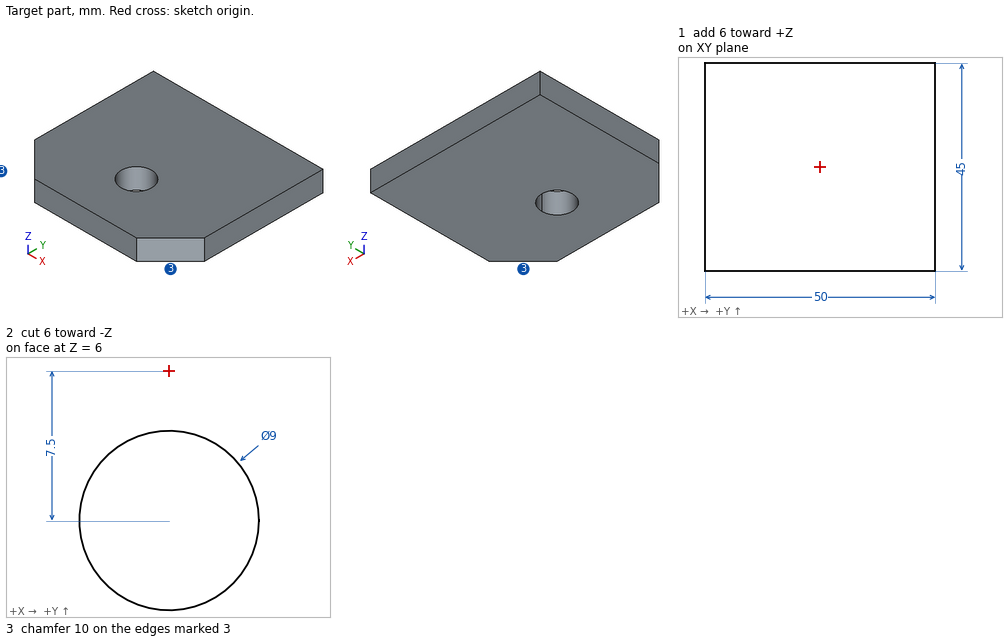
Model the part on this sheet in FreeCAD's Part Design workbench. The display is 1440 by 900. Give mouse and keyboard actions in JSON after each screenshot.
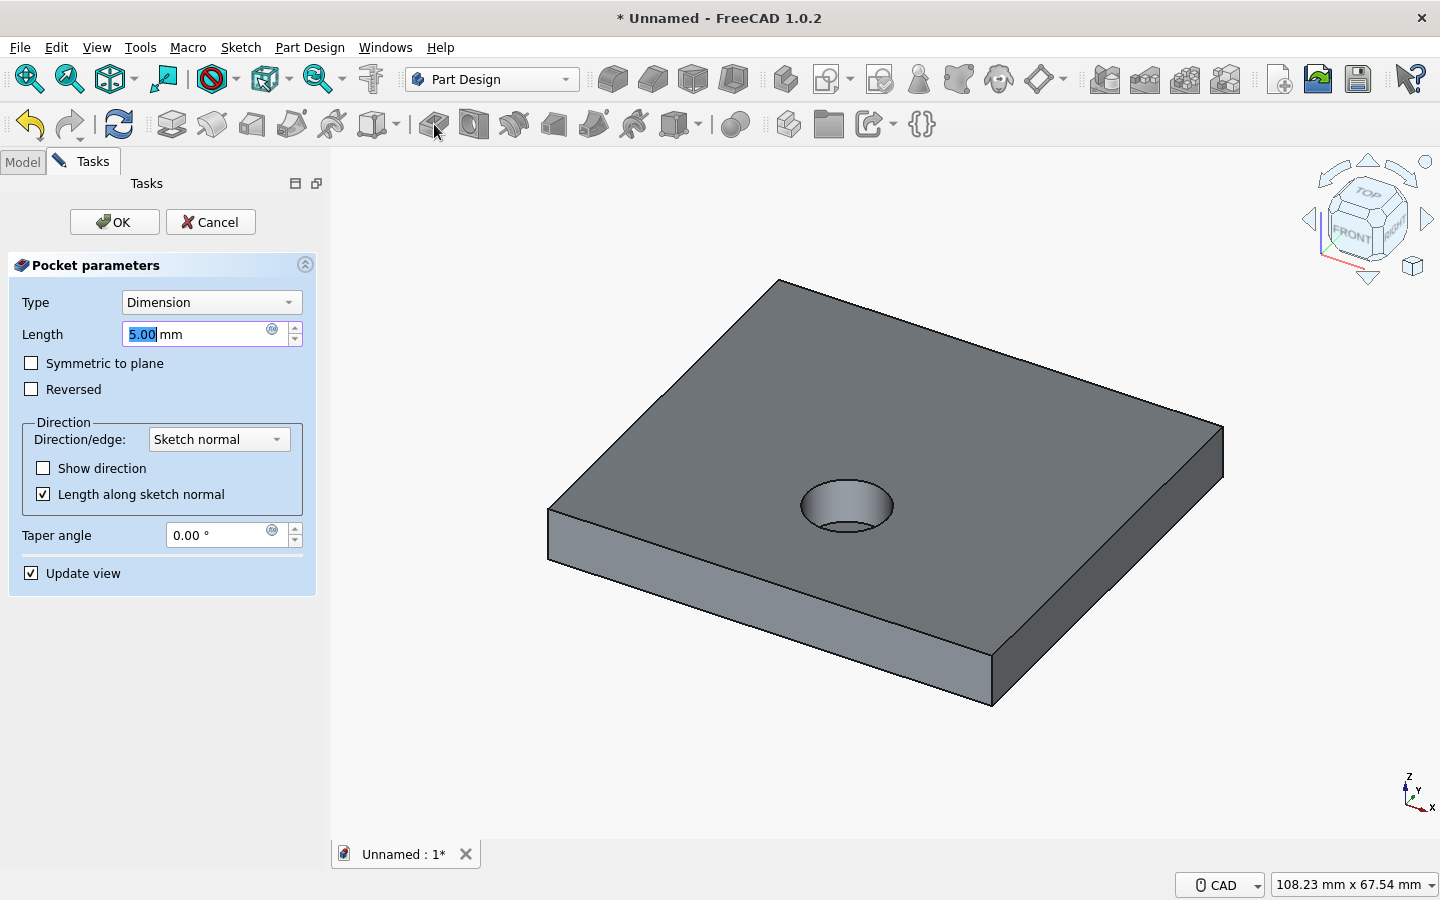
{"action": "type", "text": "6"}
{"action": "key", "text": "Tab"}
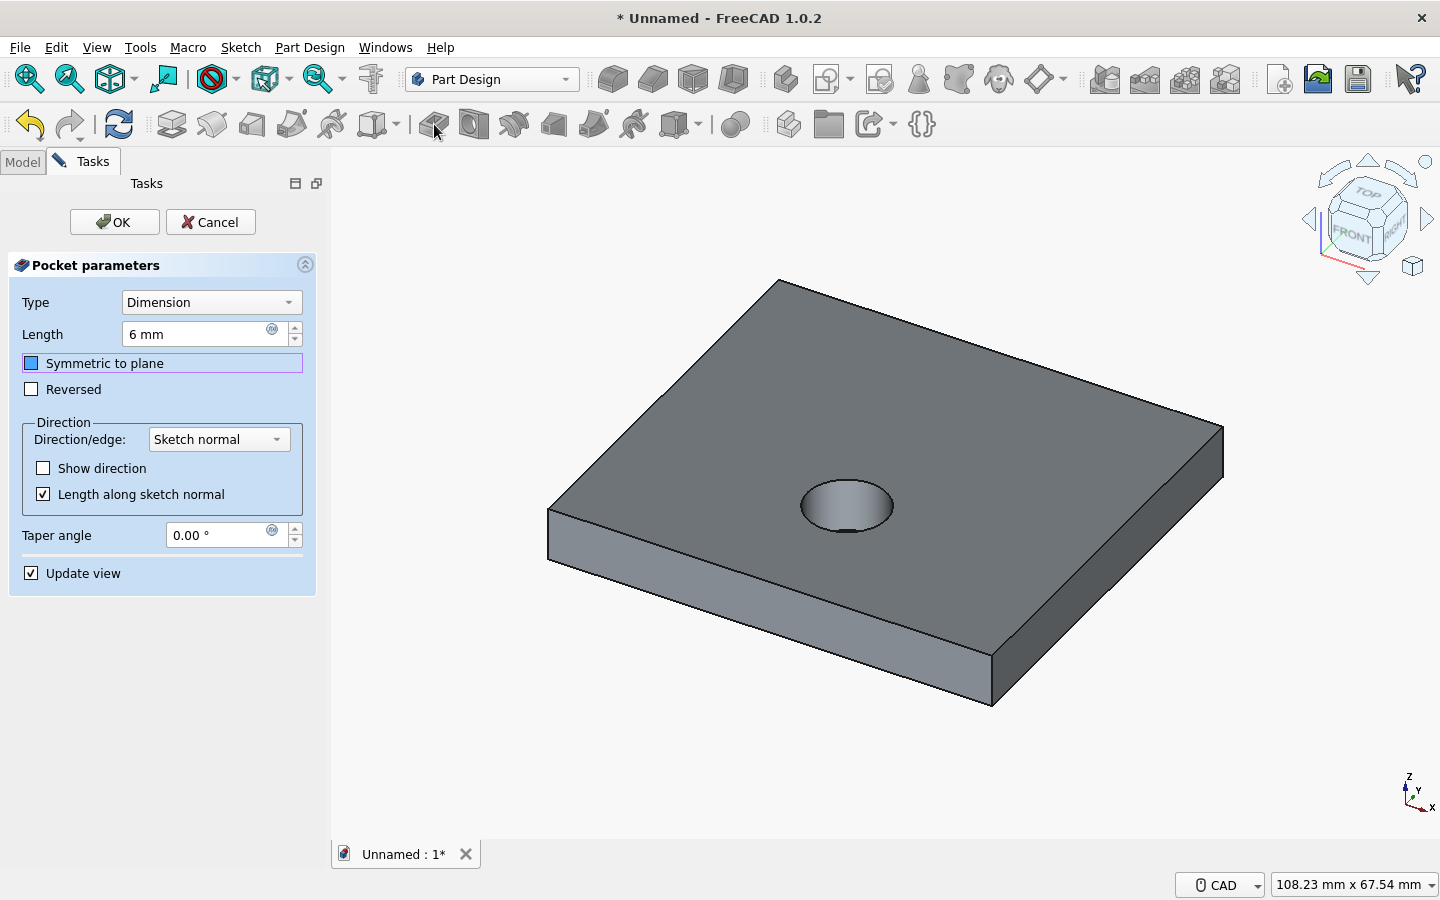
{"action": "left_click", "coordinate": [115, 222]}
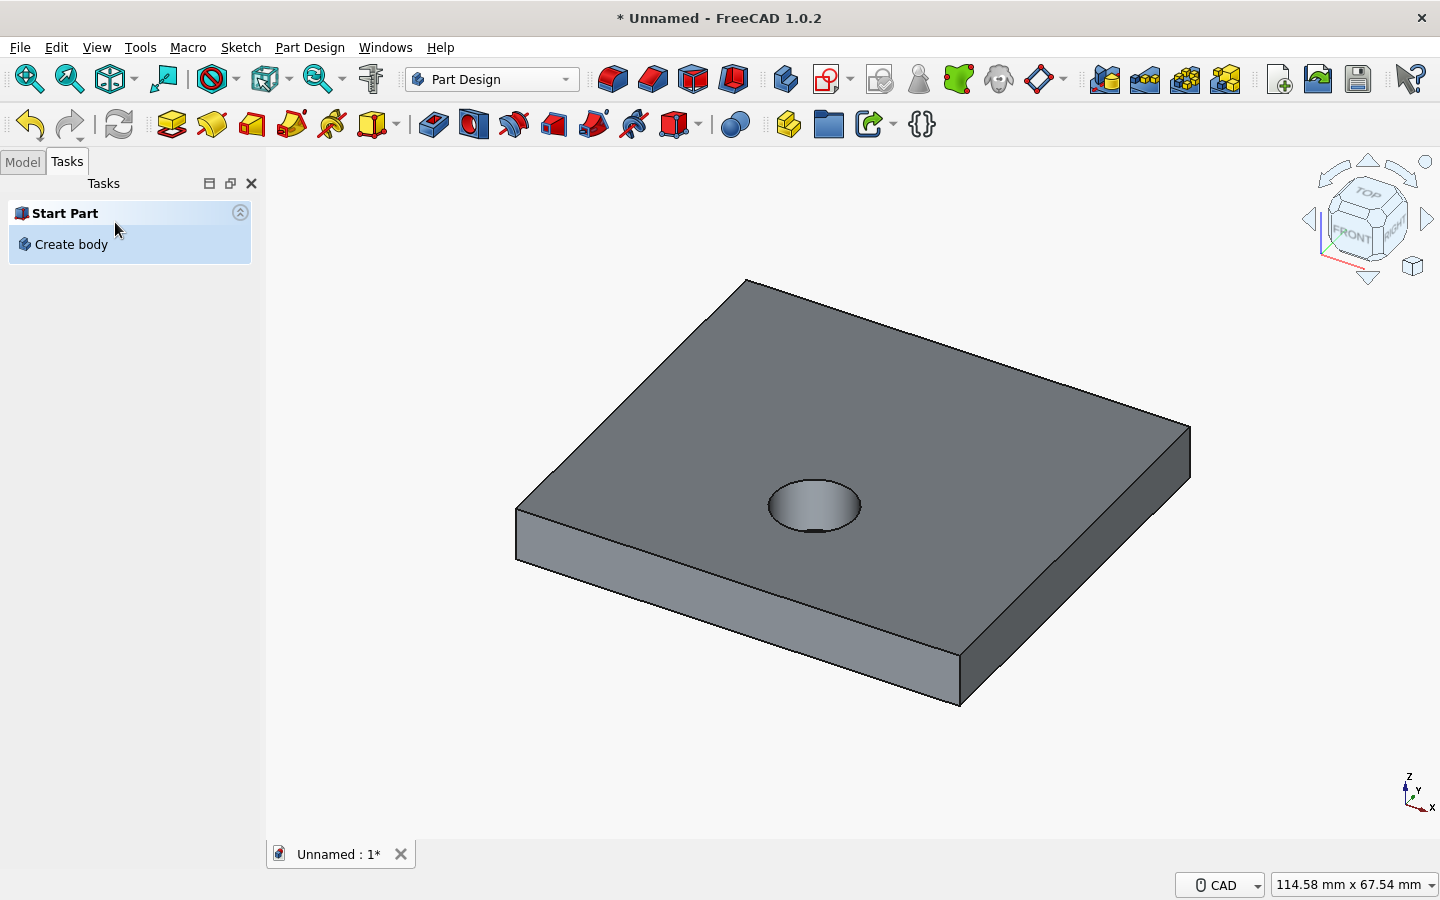
{"action": "left_click", "coordinate": [960, 680]}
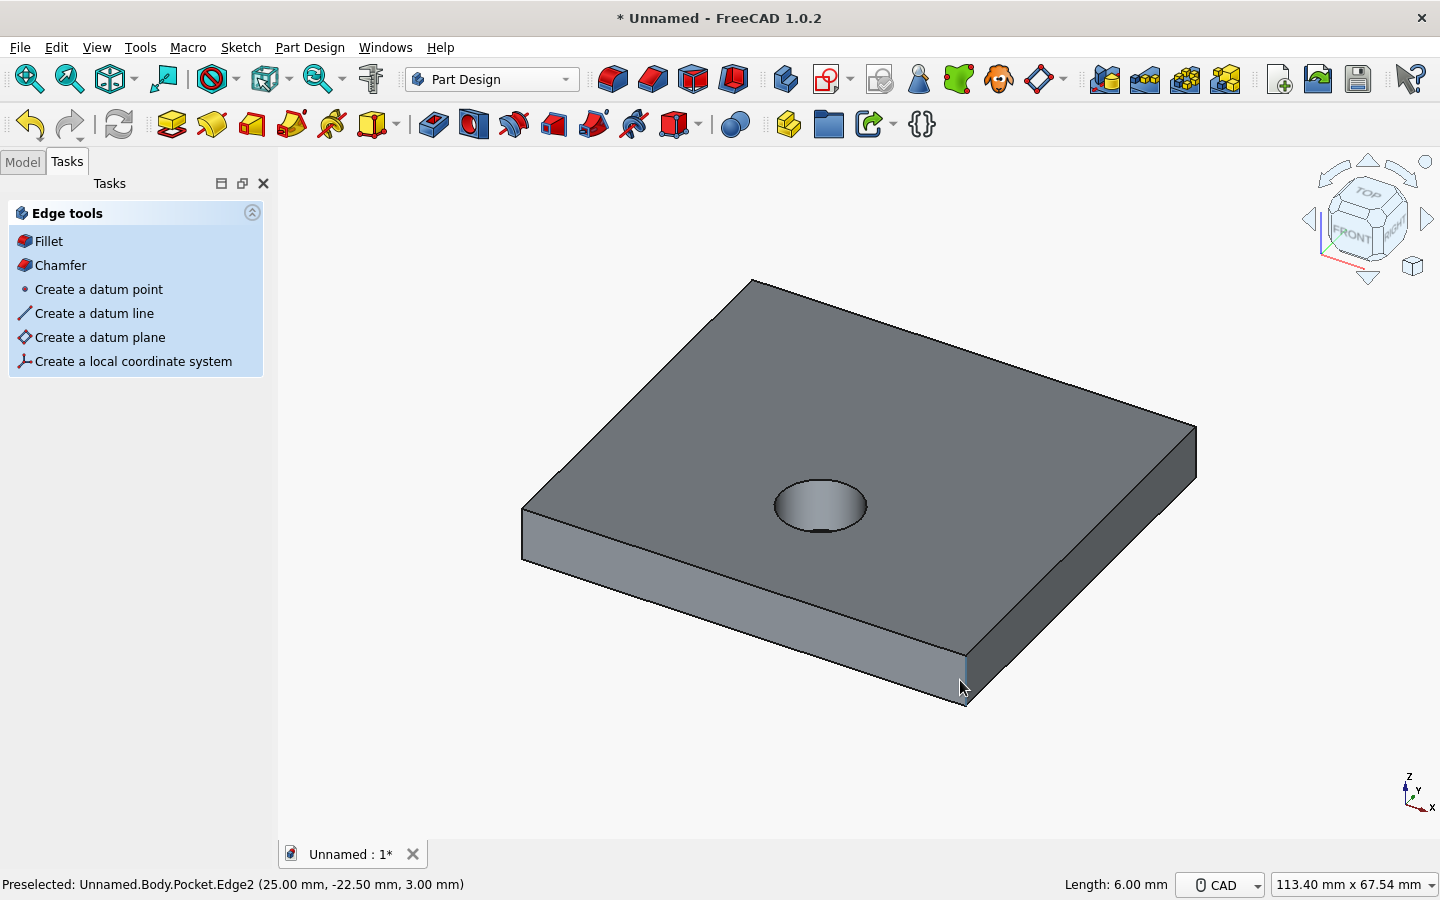
{"action": "key", "text": "0"}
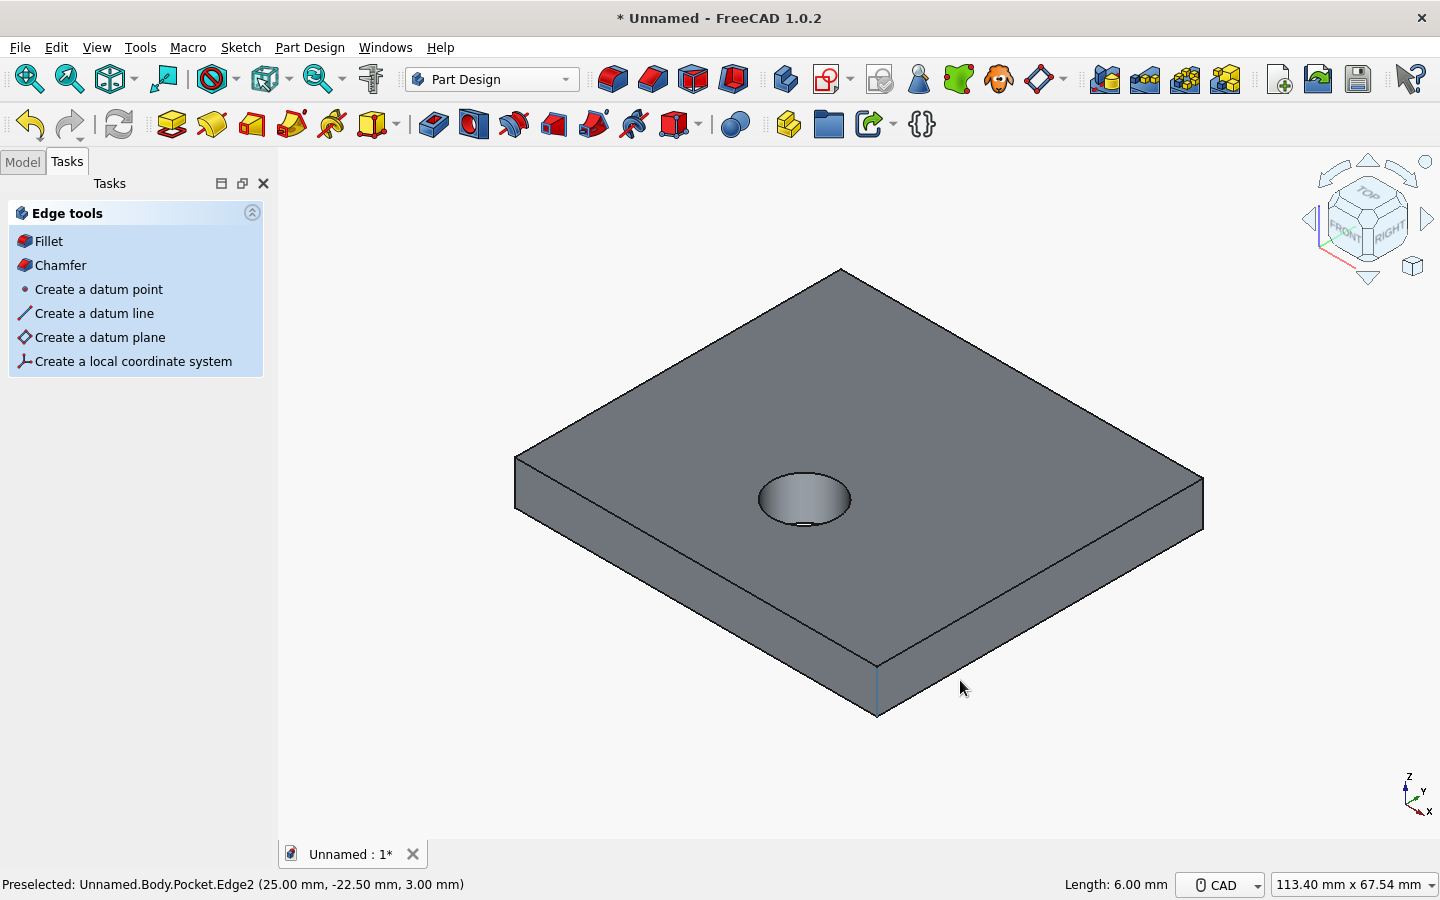
{"action": "key", "text": "2"}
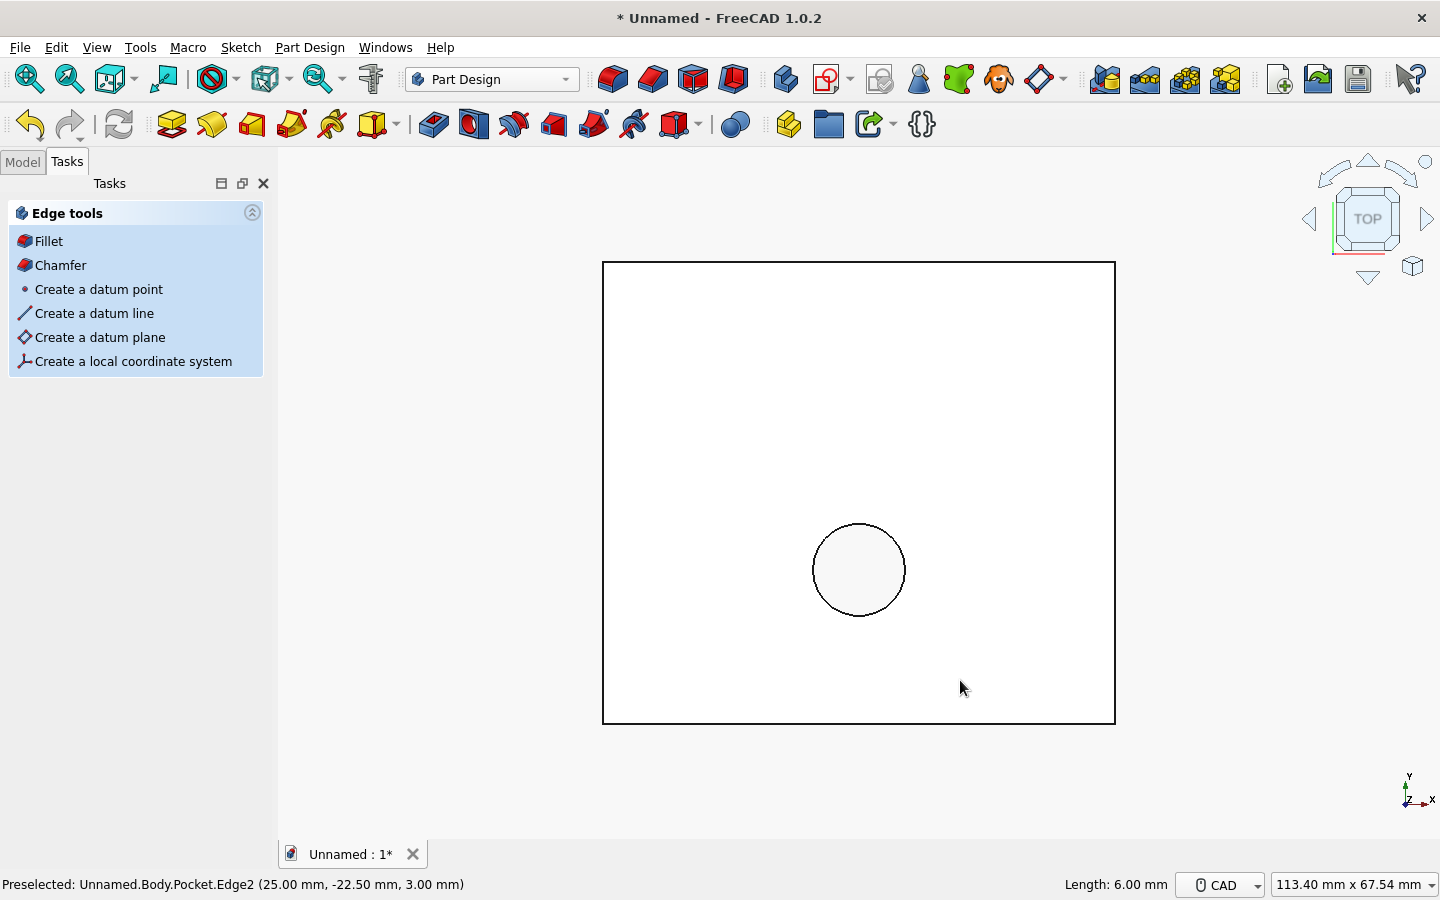
{"action": "key", "text": "1"}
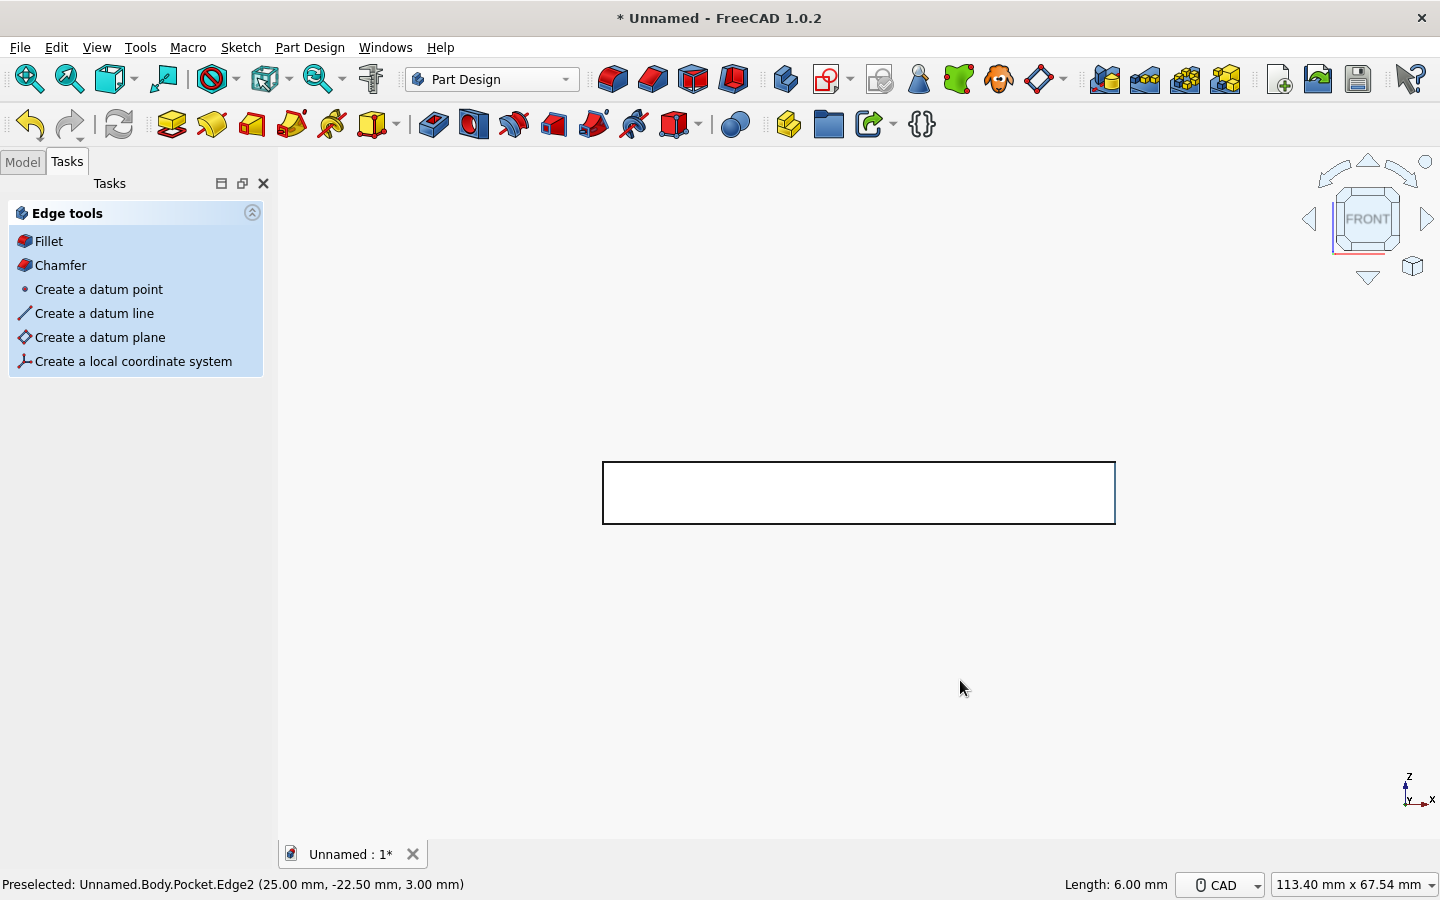
{"action": "key", "text": "v f"}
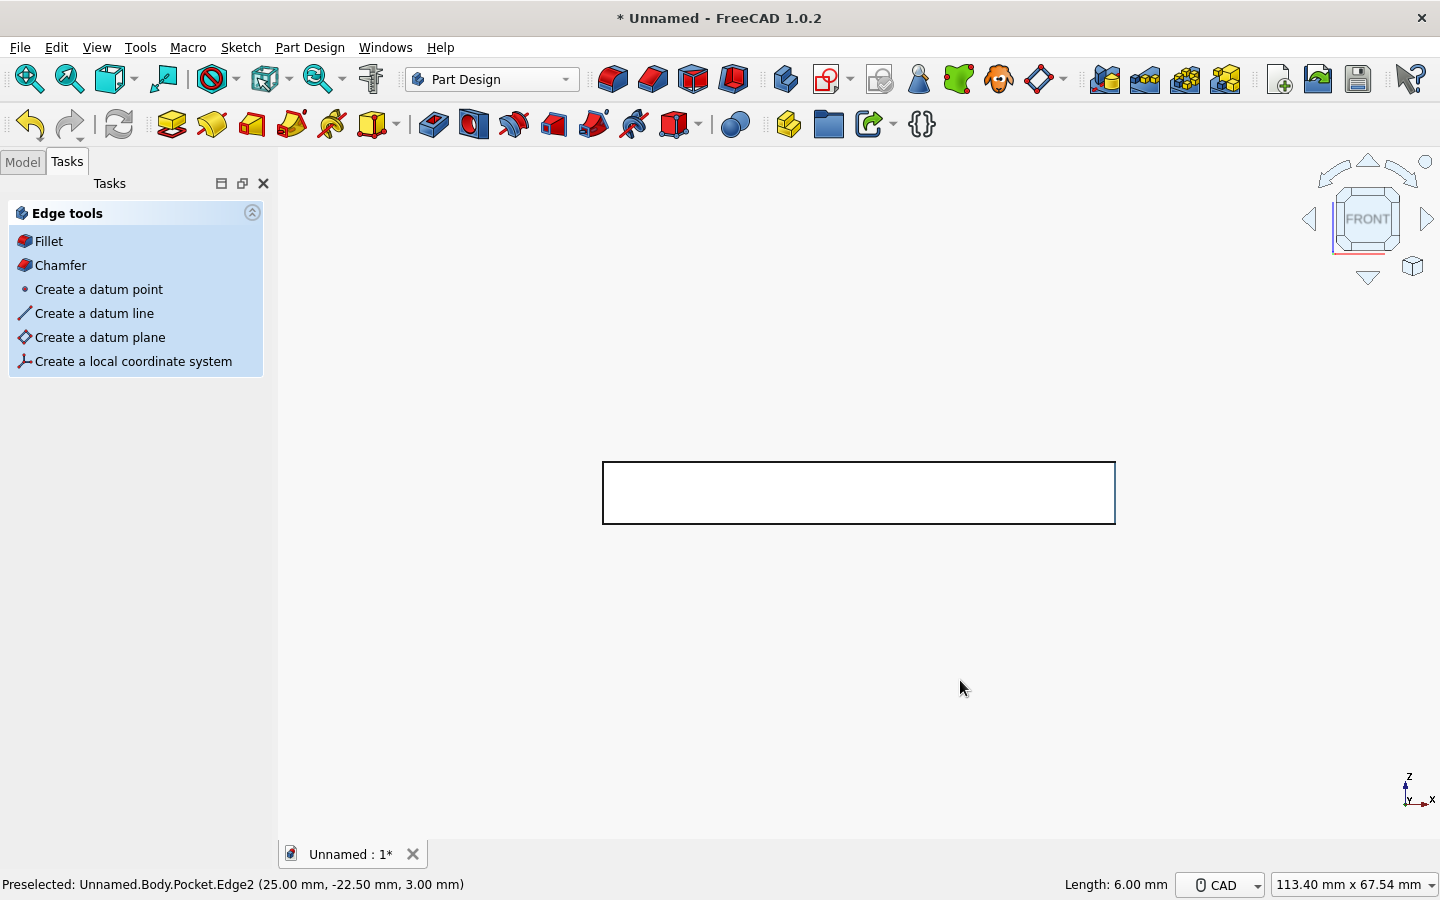
{"action": "left_click", "coordinate": [603, 492], "text": "ctrl"}